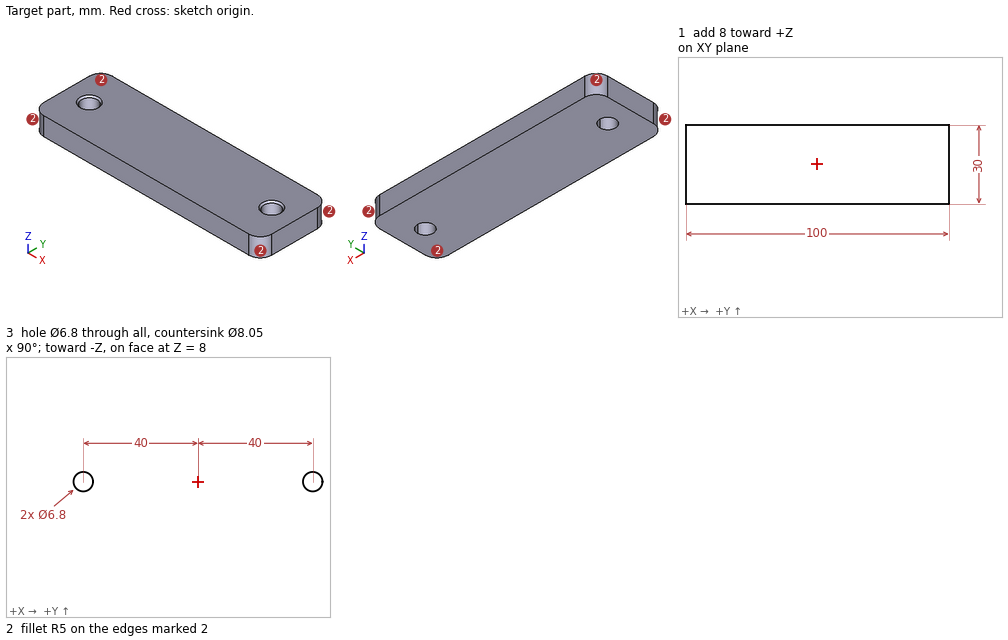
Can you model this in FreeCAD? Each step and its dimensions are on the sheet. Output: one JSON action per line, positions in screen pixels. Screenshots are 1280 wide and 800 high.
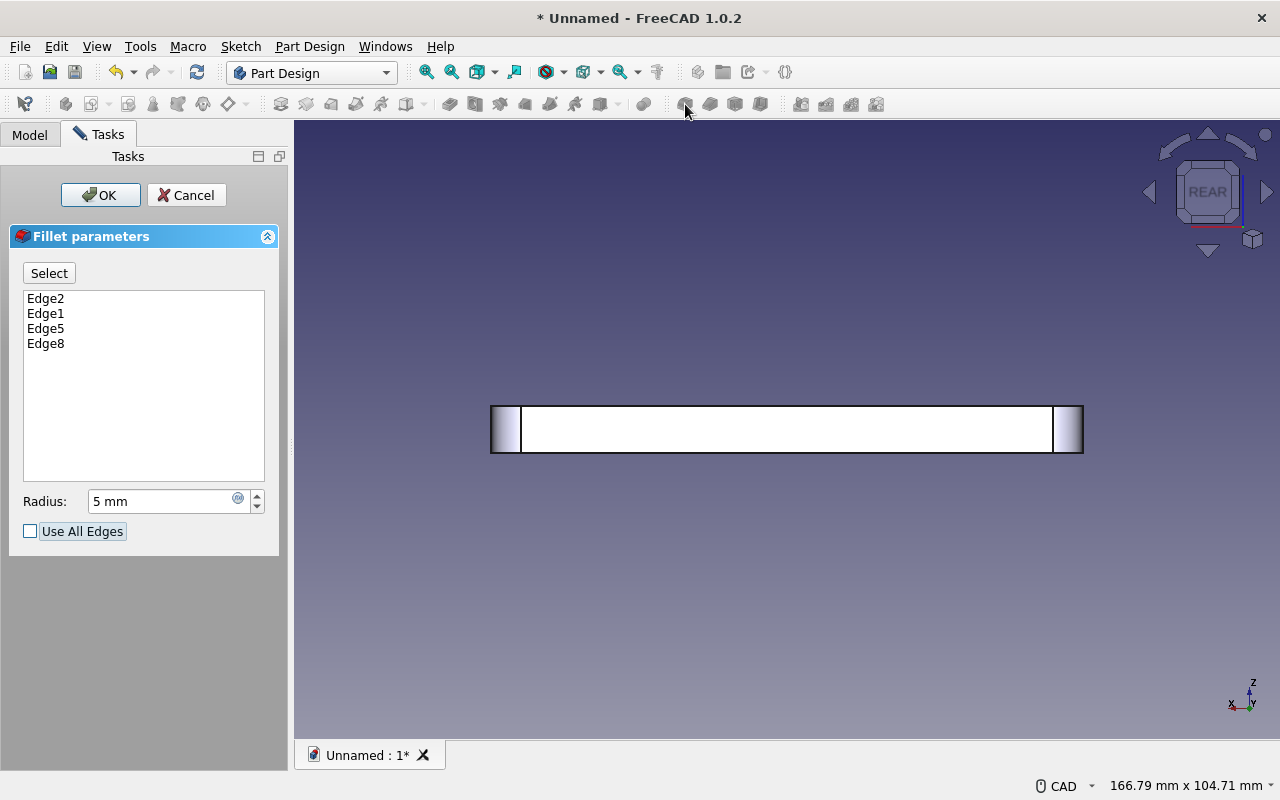
{"action": "left_click", "coordinate": [101, 195]}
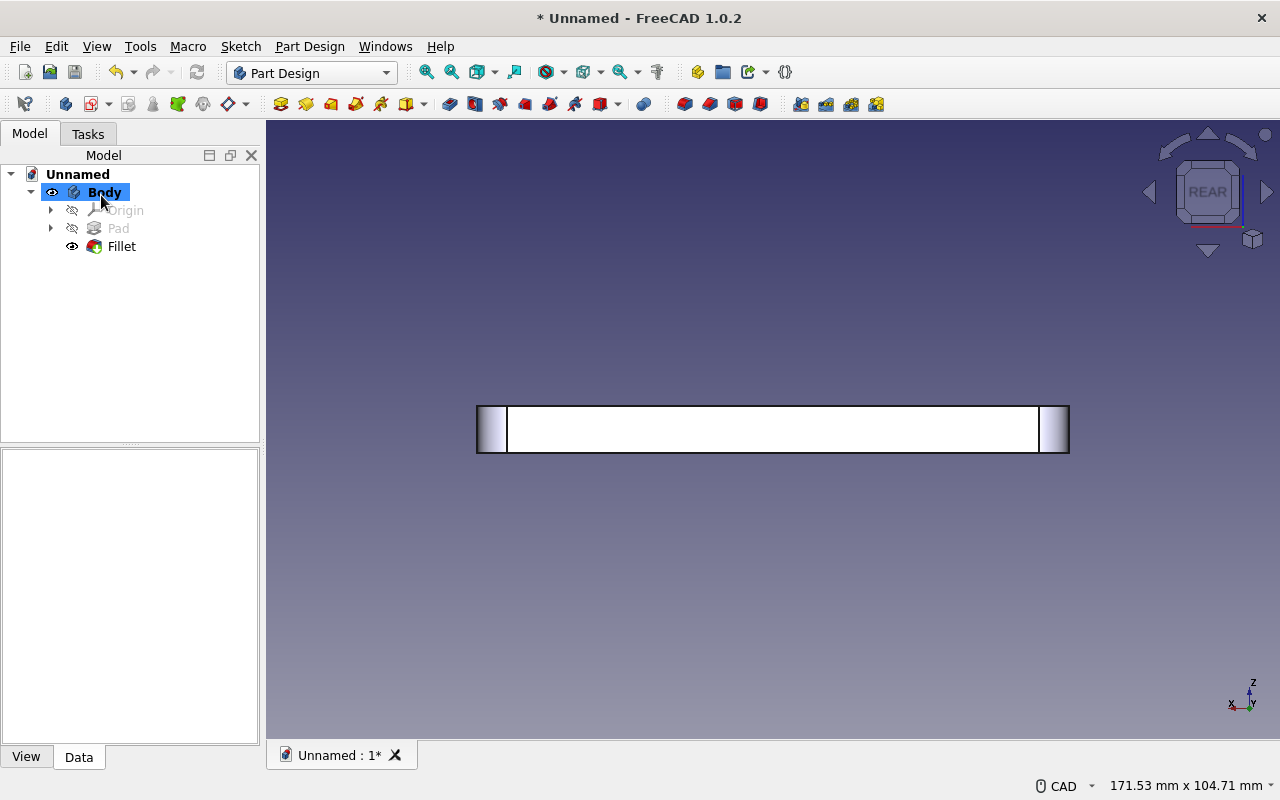
{"action": "key", "text": "0"}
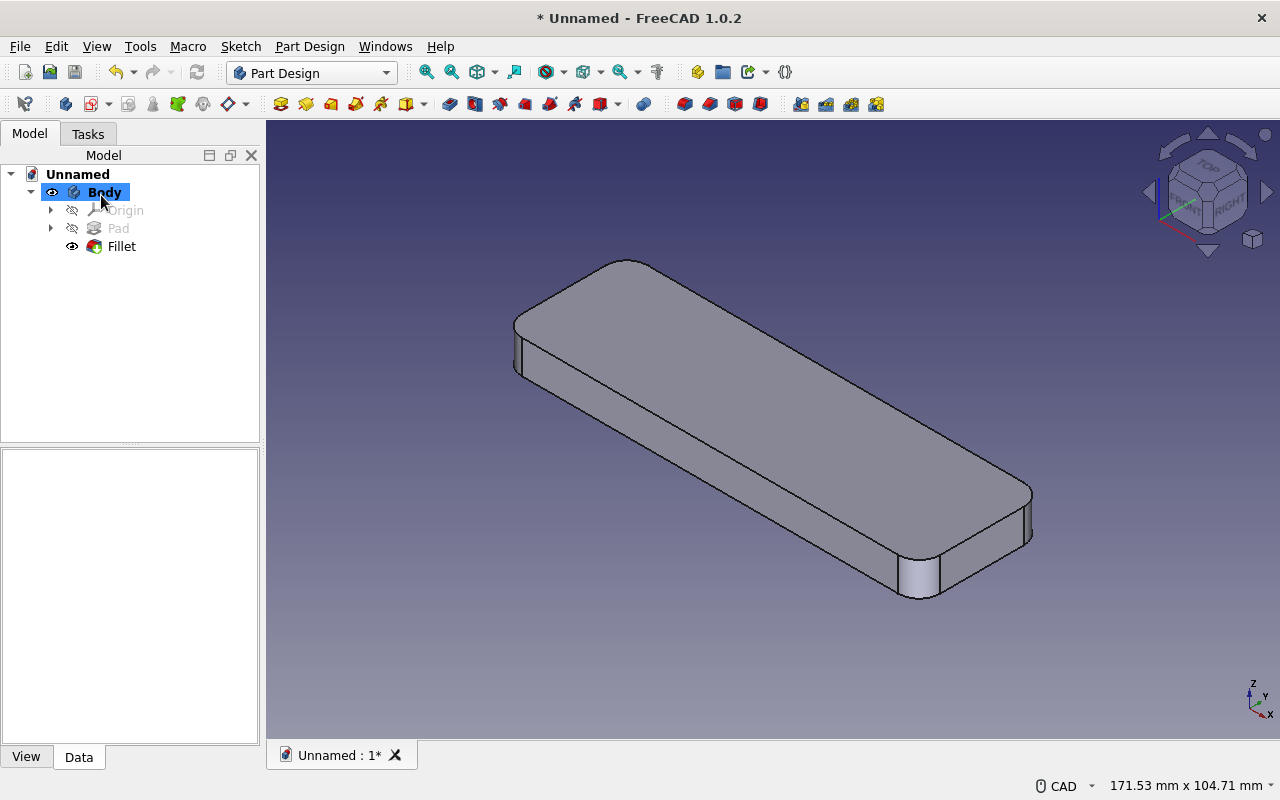
{"action": "left_click", "coordinate": [892, 478]}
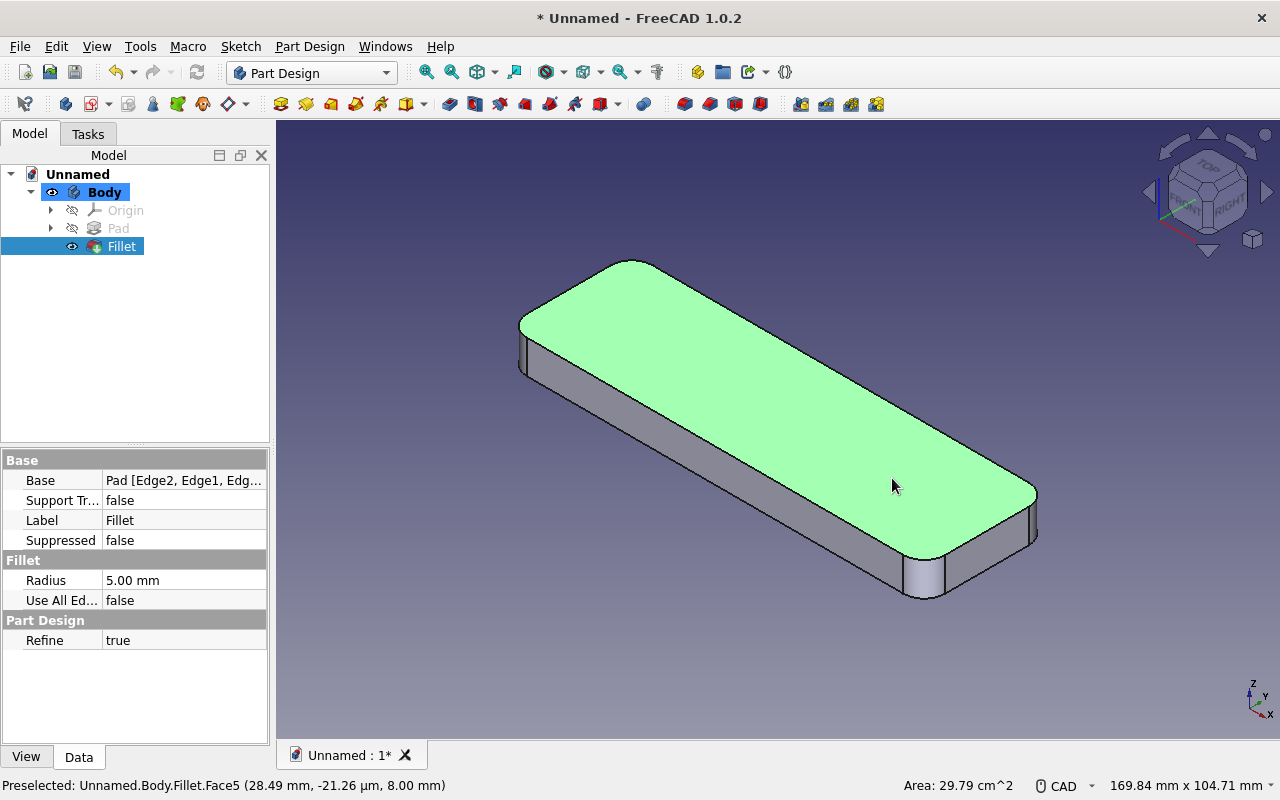
{"action": "left_click", "coordinate": [90, 104]}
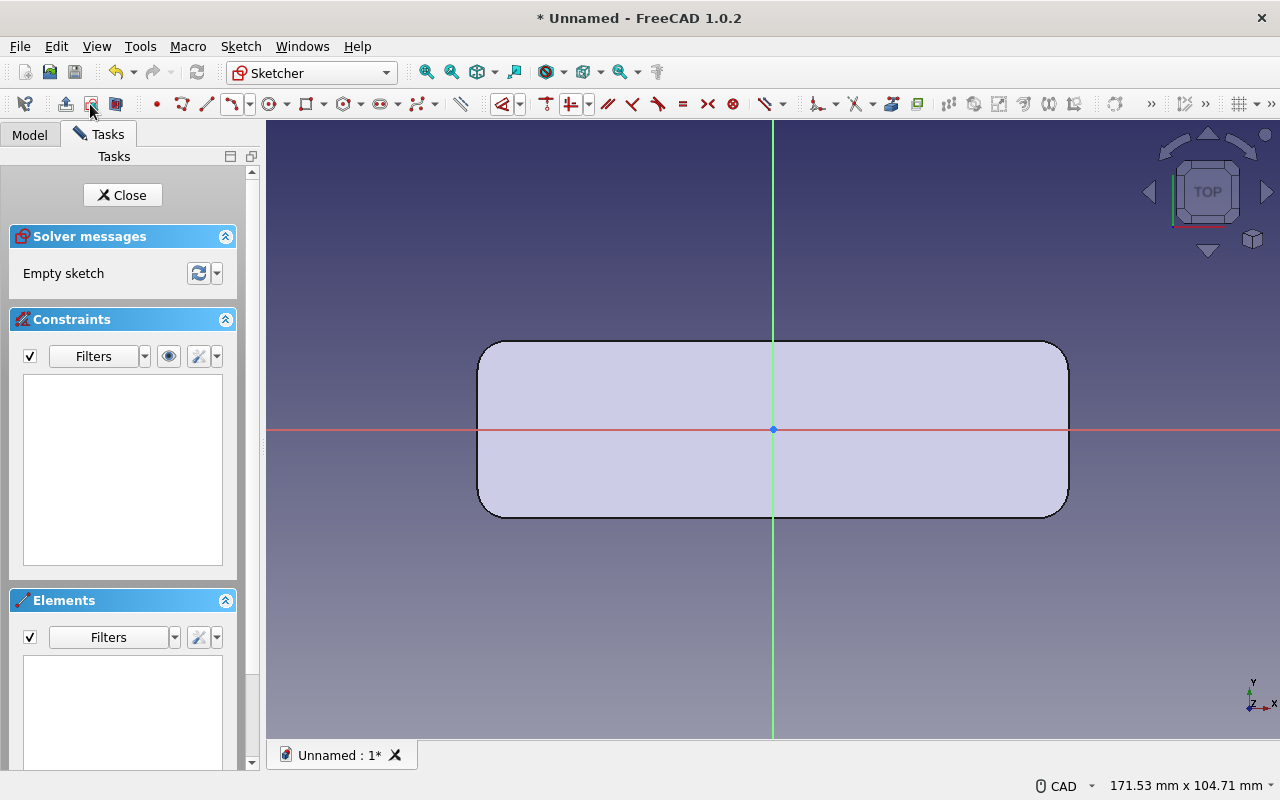
{"action": "left_click", "coordinate": [268, 104]}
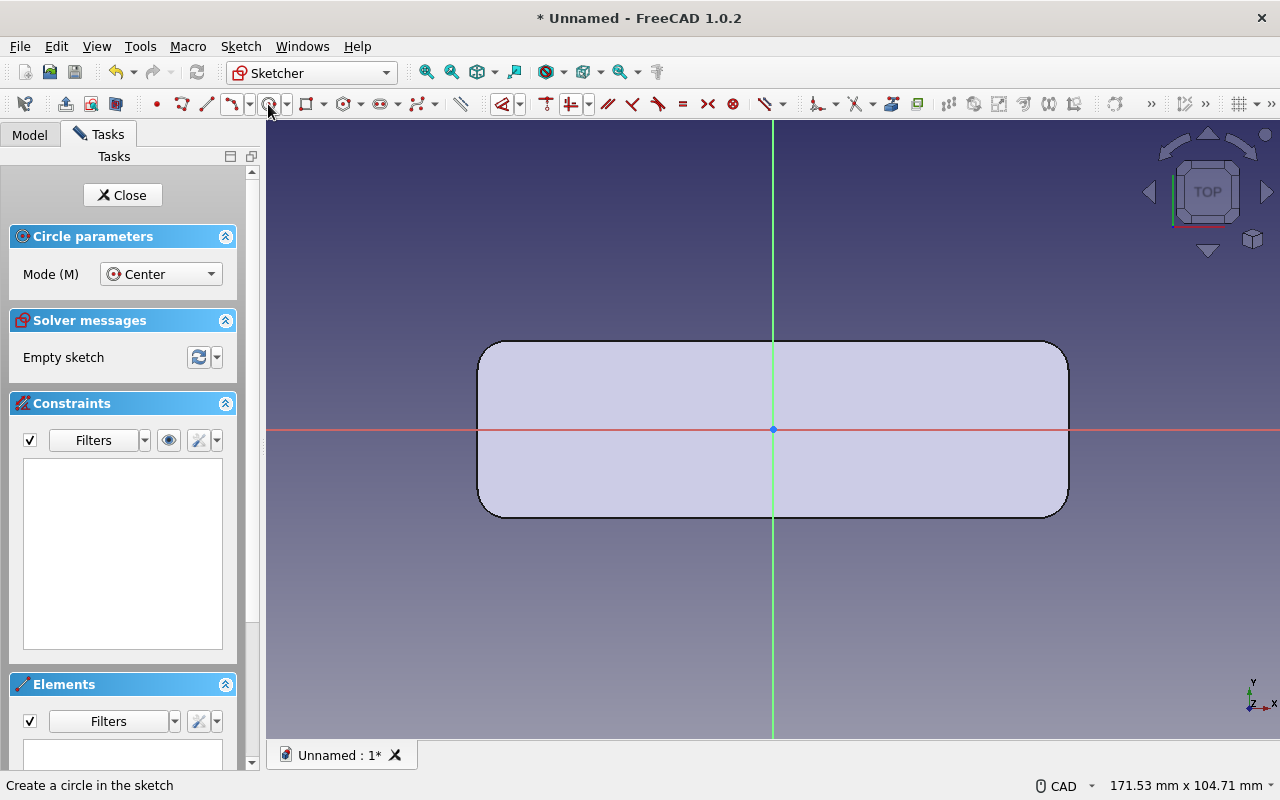
{"action": "left_click", "coordinate": [537, 430]}
{"action": "left_click", "coordinate": [551, 415]}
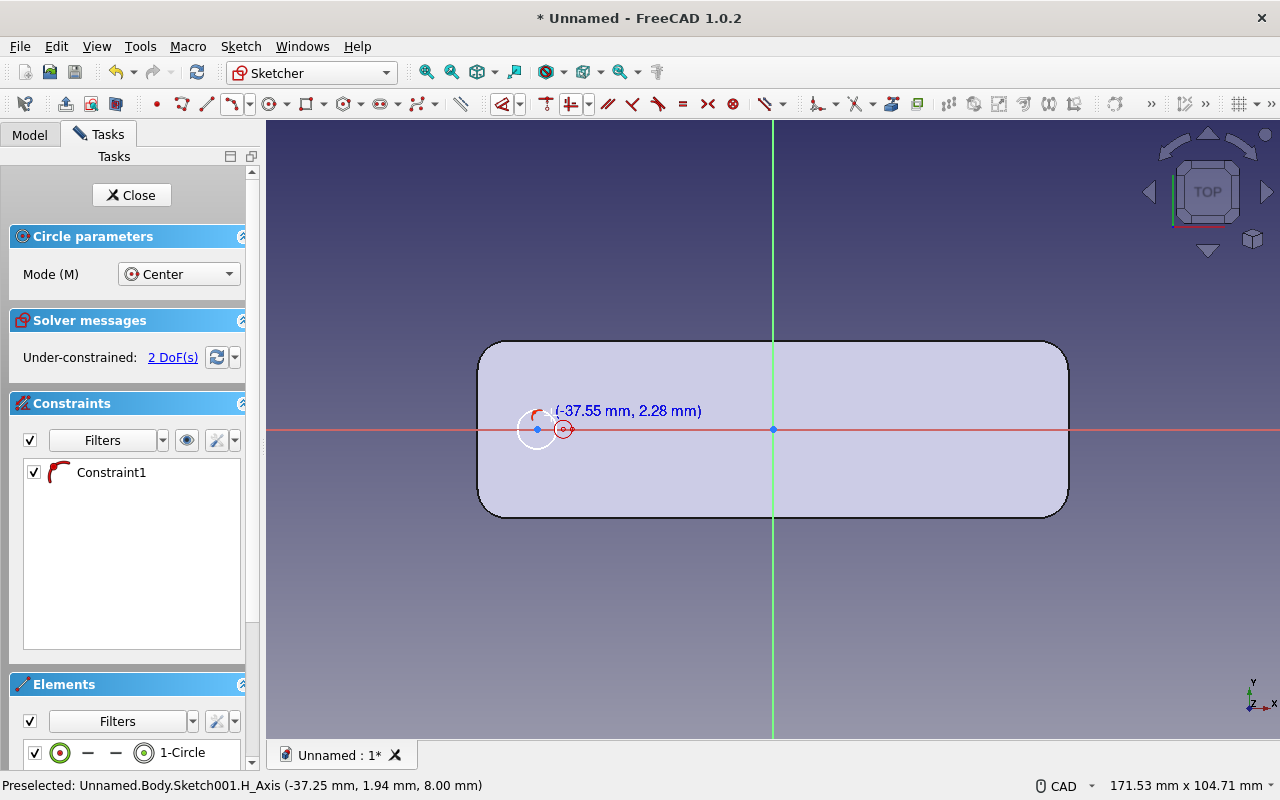
{"action": "left_click", "coordinate": [1009, 430]}
{"action": "left_click", "coordinate": [1024, 415]}
{"action": "key", "text": "Escape"}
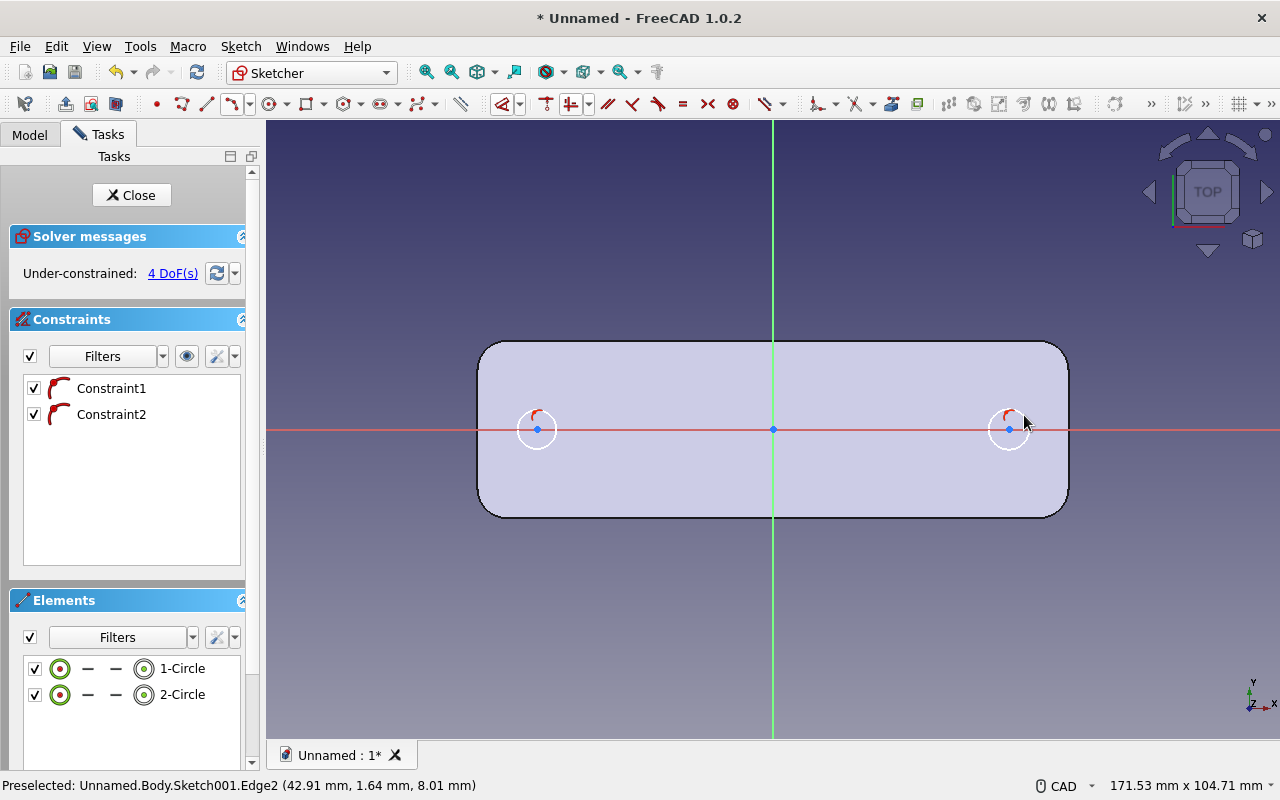
{"action": "left_click", "coordinate": [551, 416]}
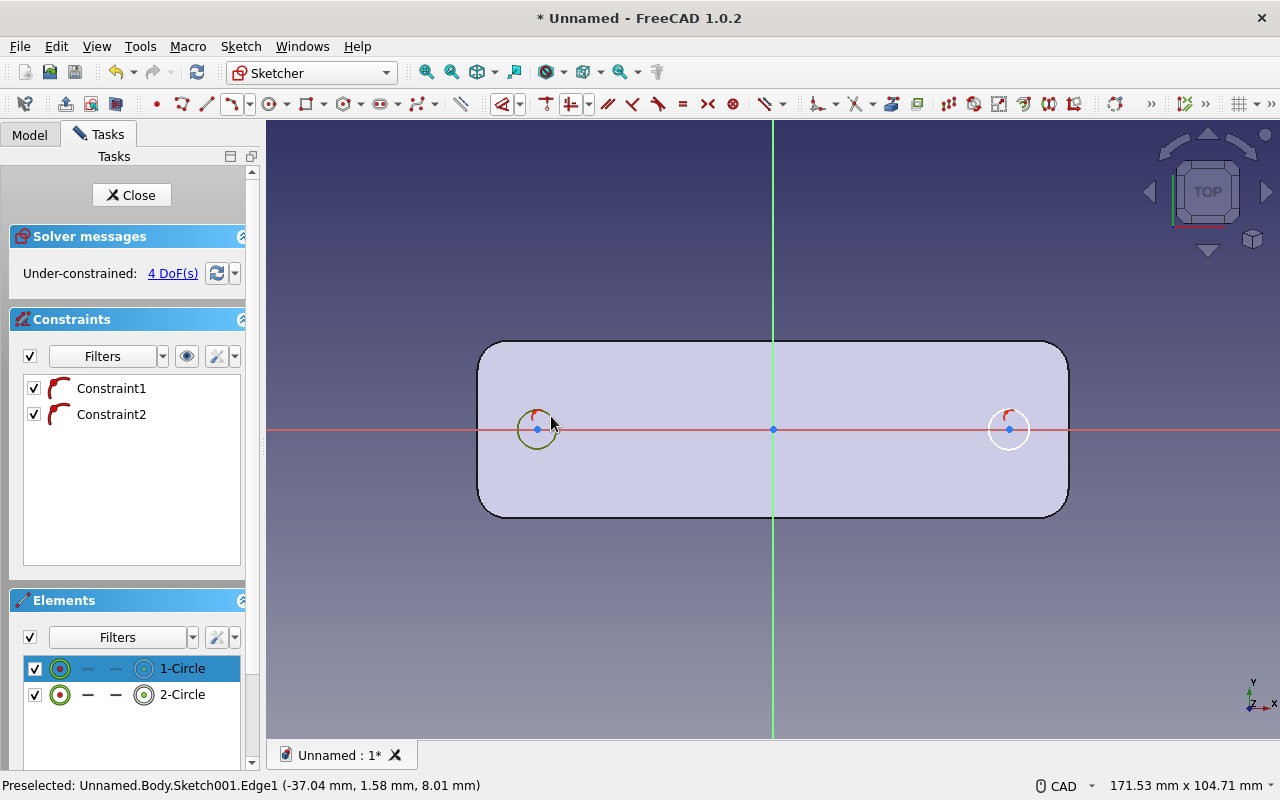
{"action": "left_click", "coordinate": [1023, 415]}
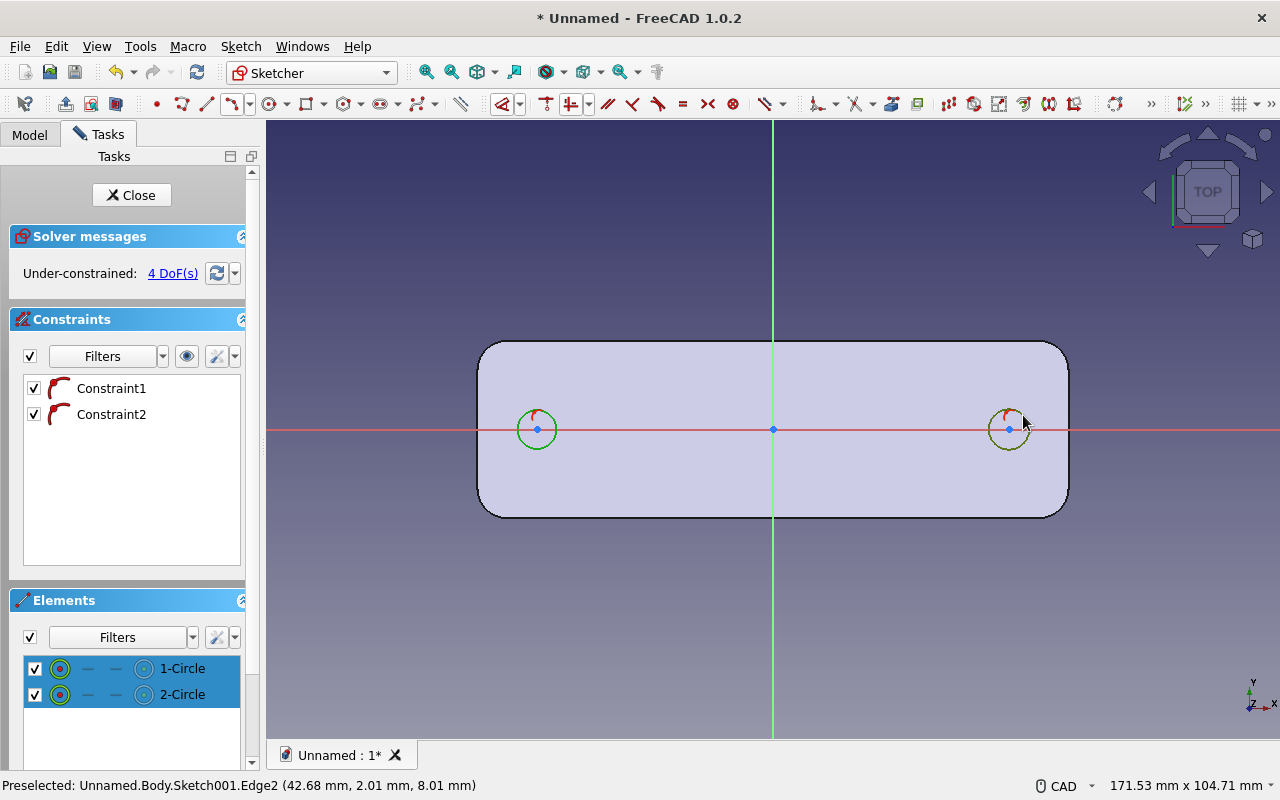
{"action": "left_click", "coordinate": [683, 104]}